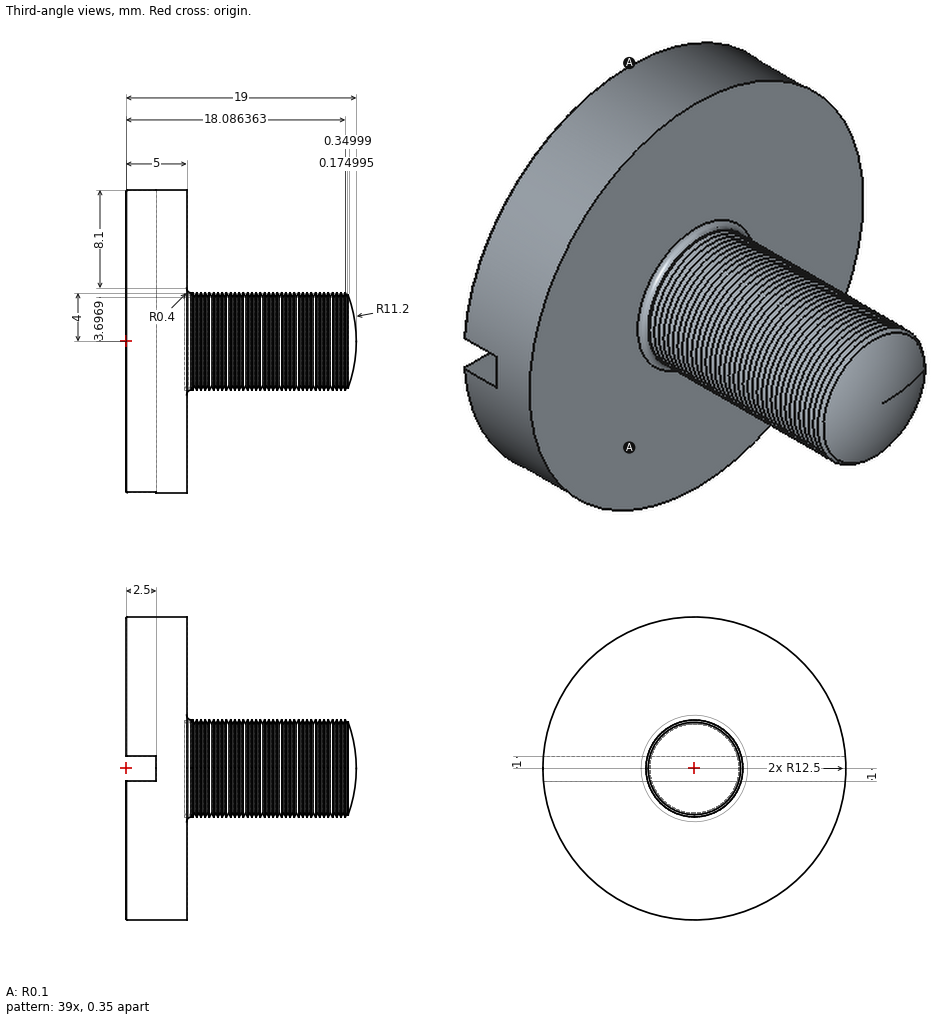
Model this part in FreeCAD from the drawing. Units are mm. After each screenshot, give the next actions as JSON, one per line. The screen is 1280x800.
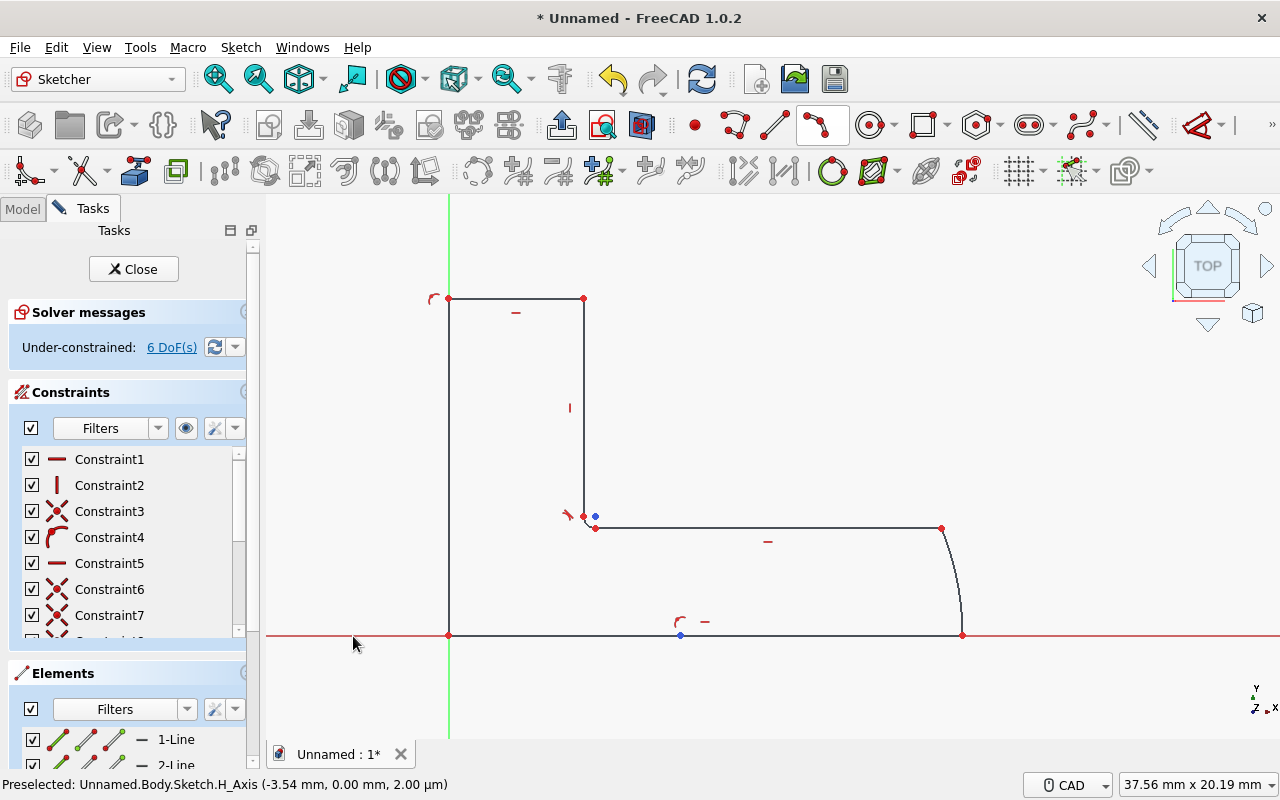
{"action": "scroll", "coordinate": [587, 525], "scroll_direction": "up", "scroll_amount": 7}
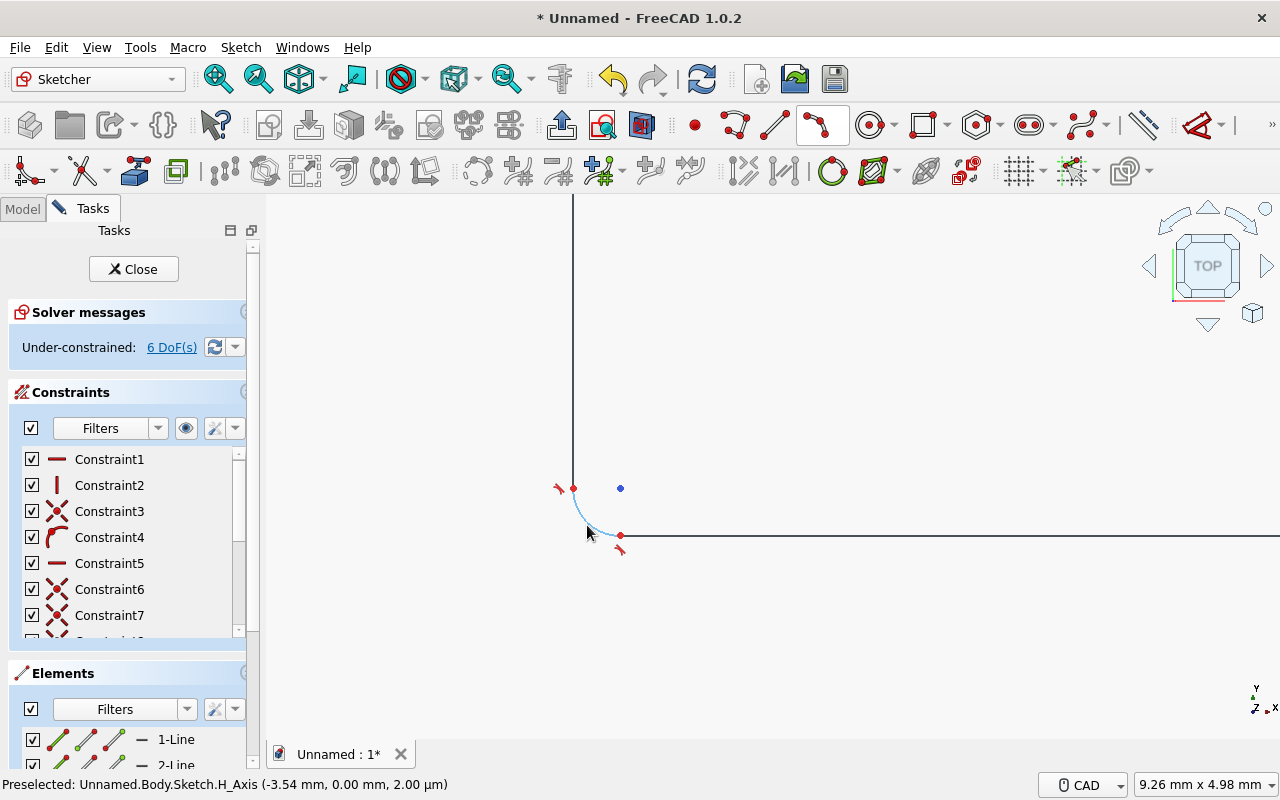
{"action": "left_click", "coordinate": [587, 522]}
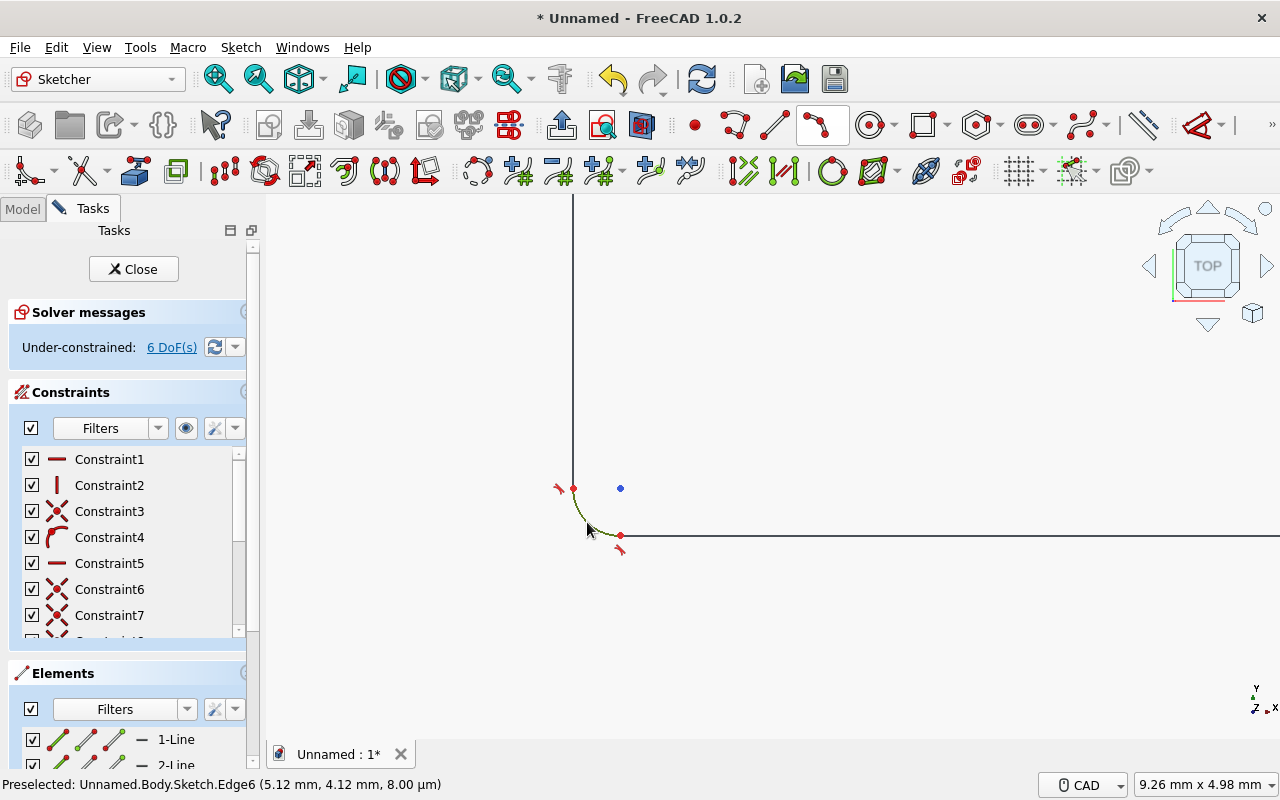
{"action": "left_click", "coordinate": [1224, 126]}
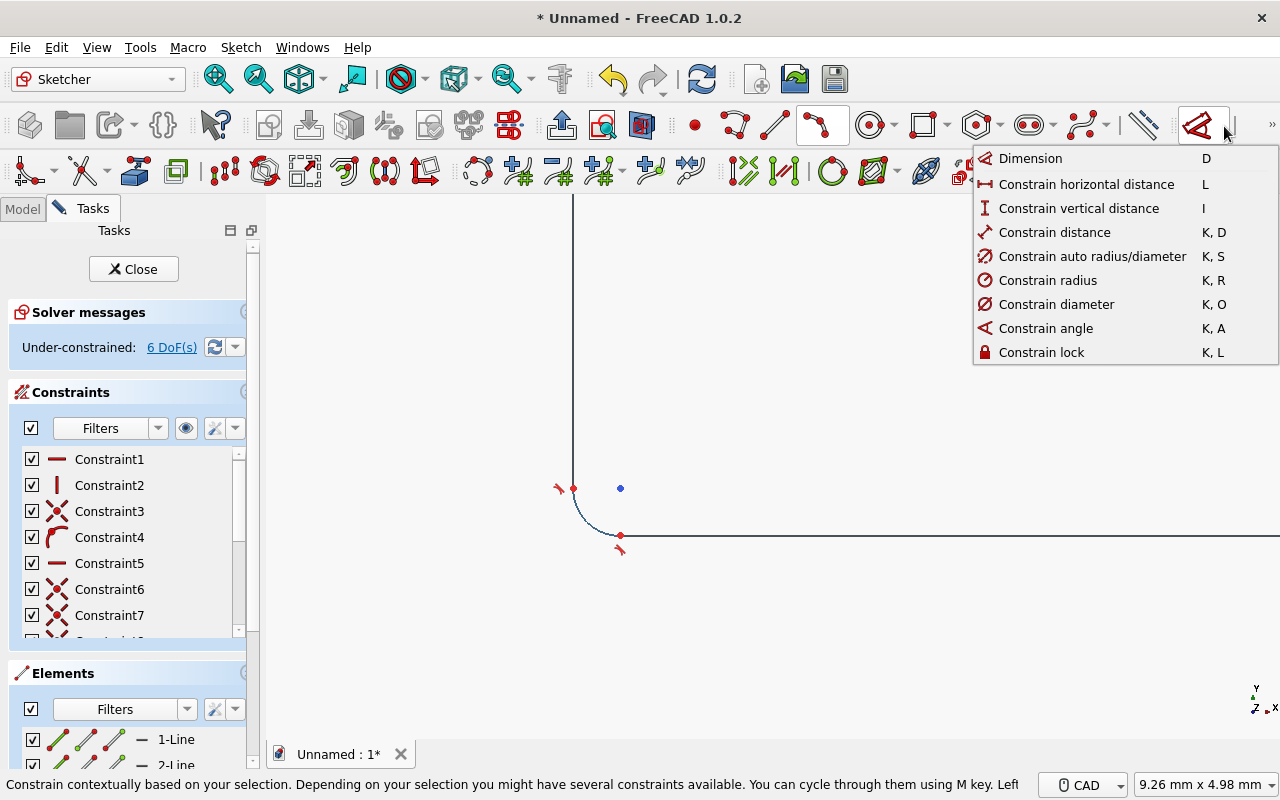
{"action": "left_click", "coordinate": [1126, 280]}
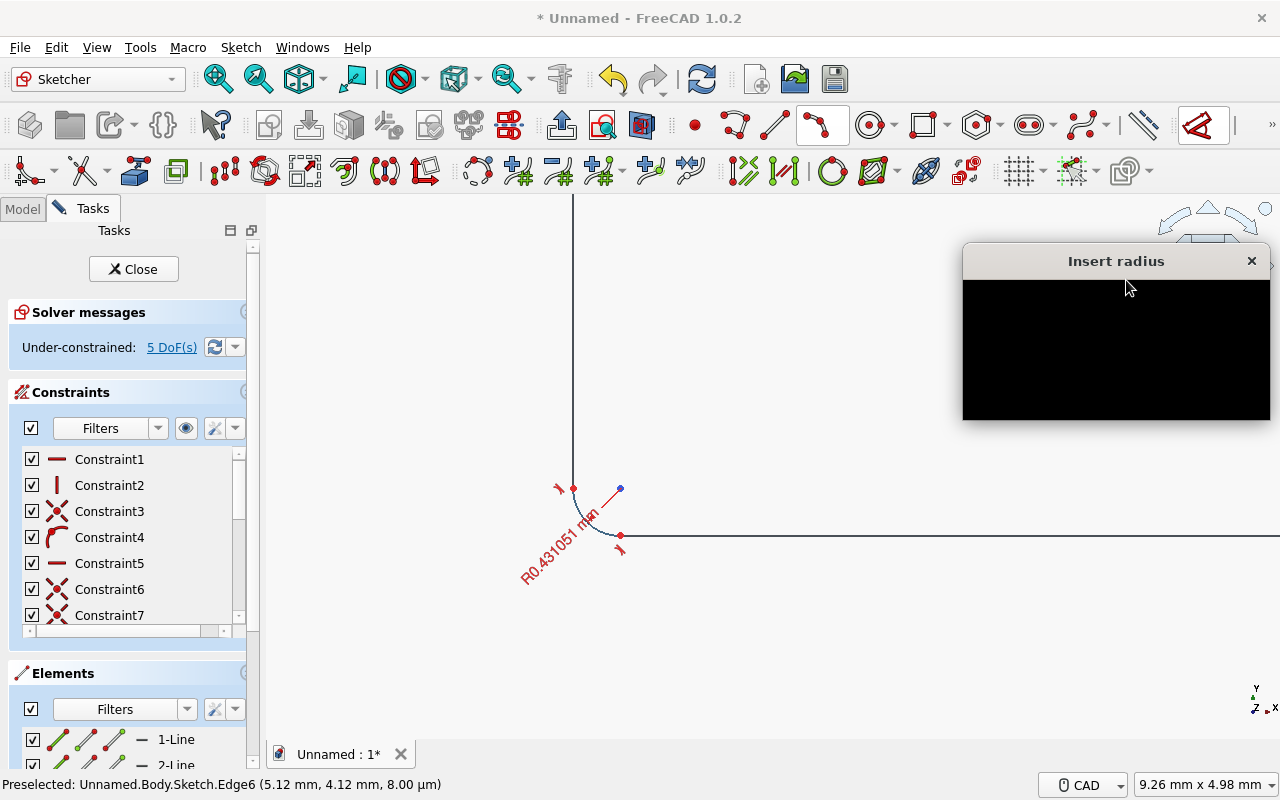
{"action": "type", "text": "0.4"}
{"action": "key", "text": "Return"}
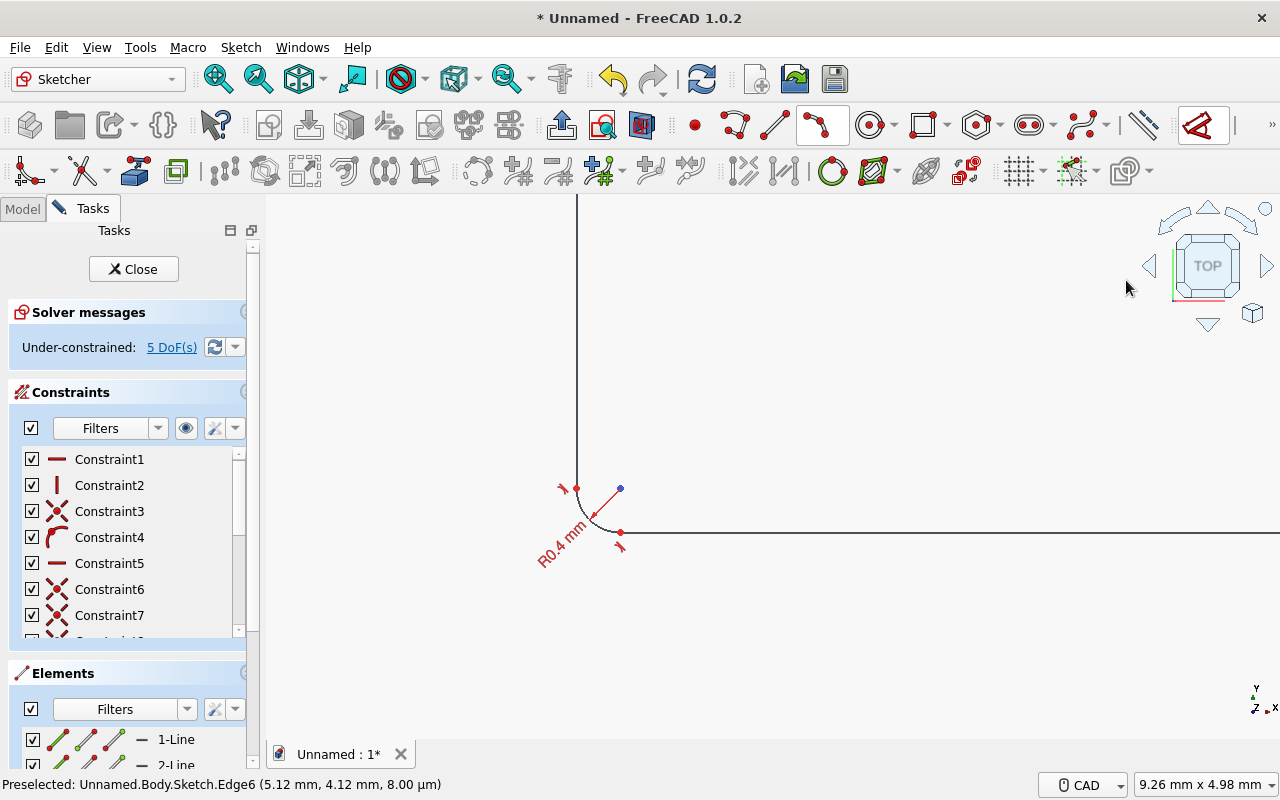
{"action": "scroll", "coordinate": [587, 525], "scroll_direction": "down", "scroll_amount": 7}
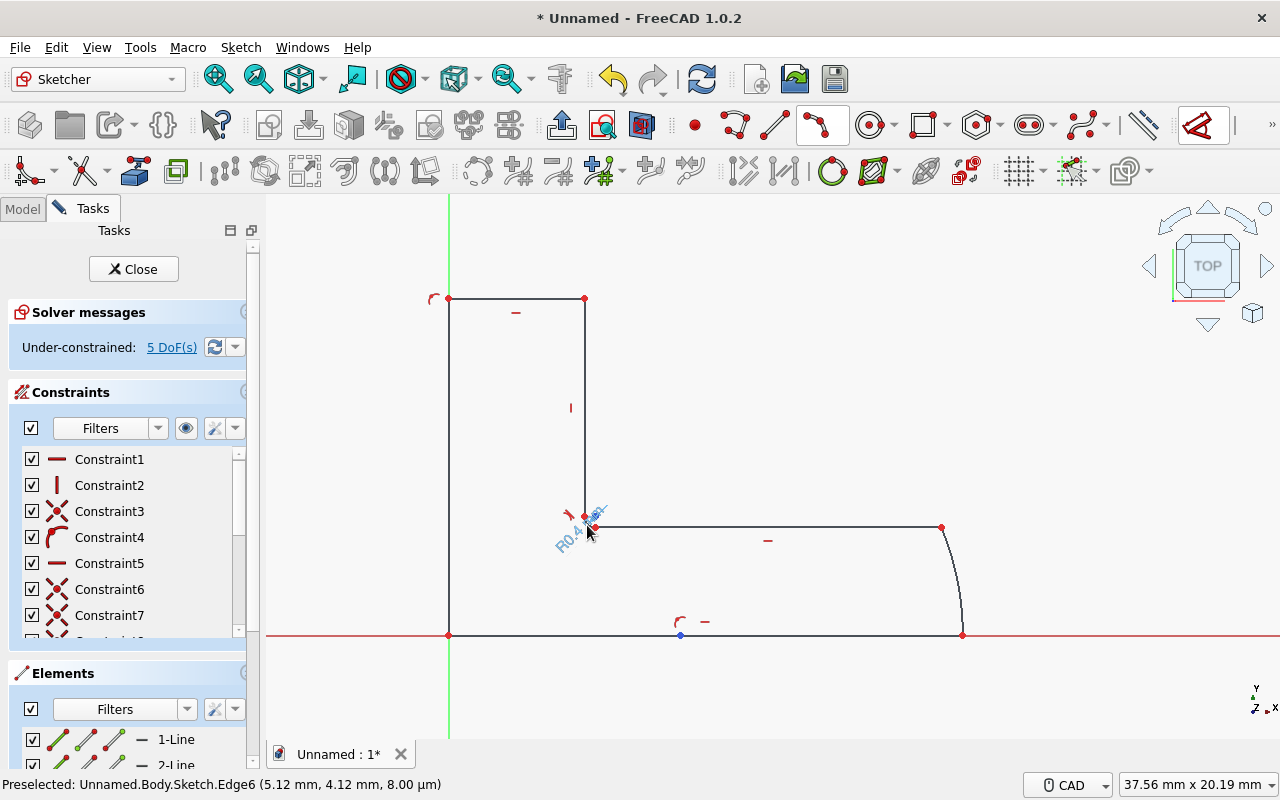
{"action": "left_click", "coordinate": [961, 602]}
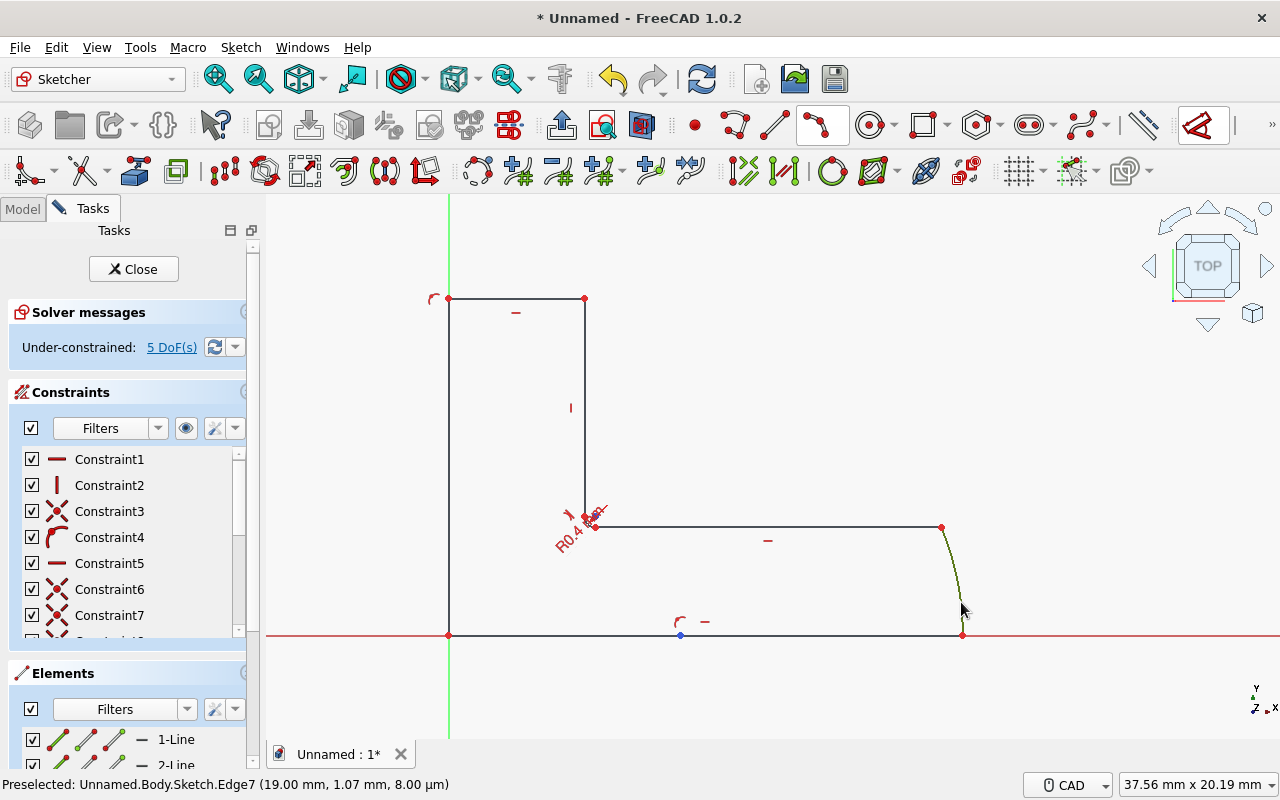
{"action": "key", "text": "k r"}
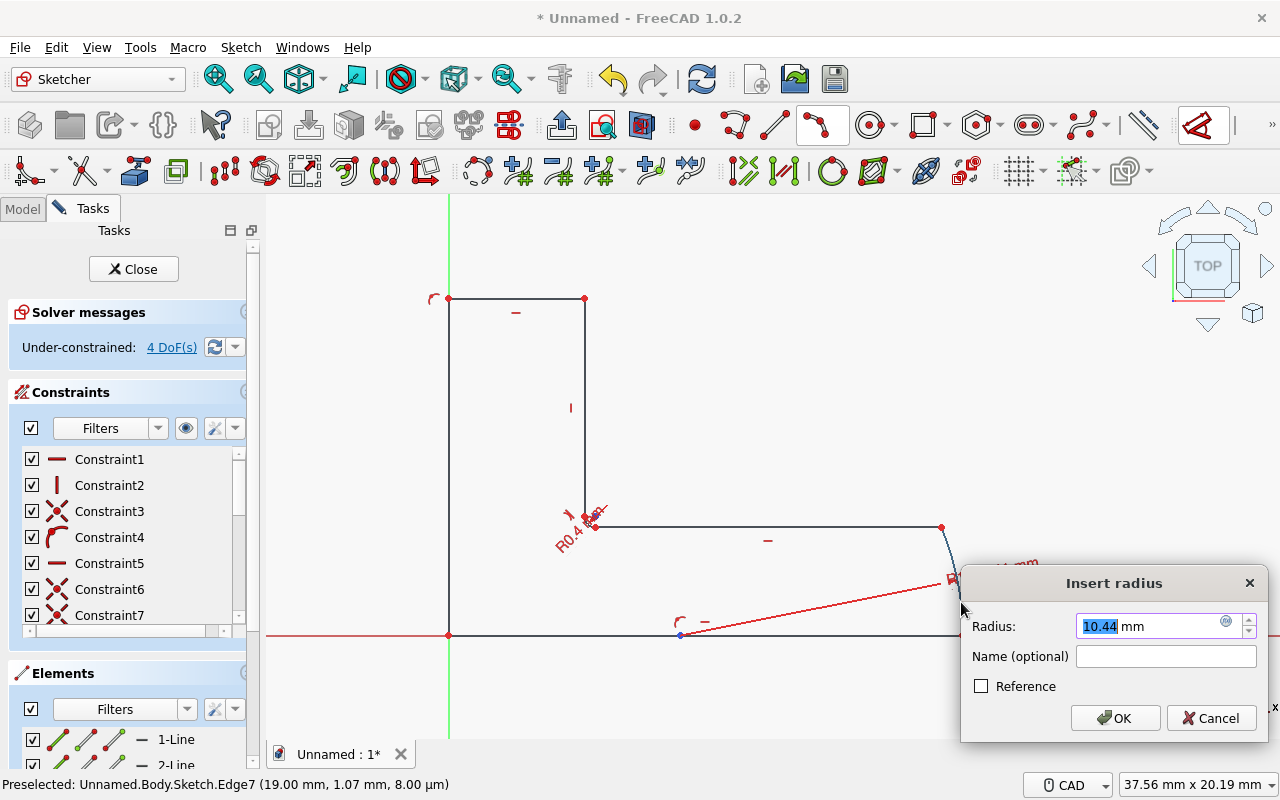
{"action": "type", "text": "11.2"}
{"action": "key", "text": "Return"}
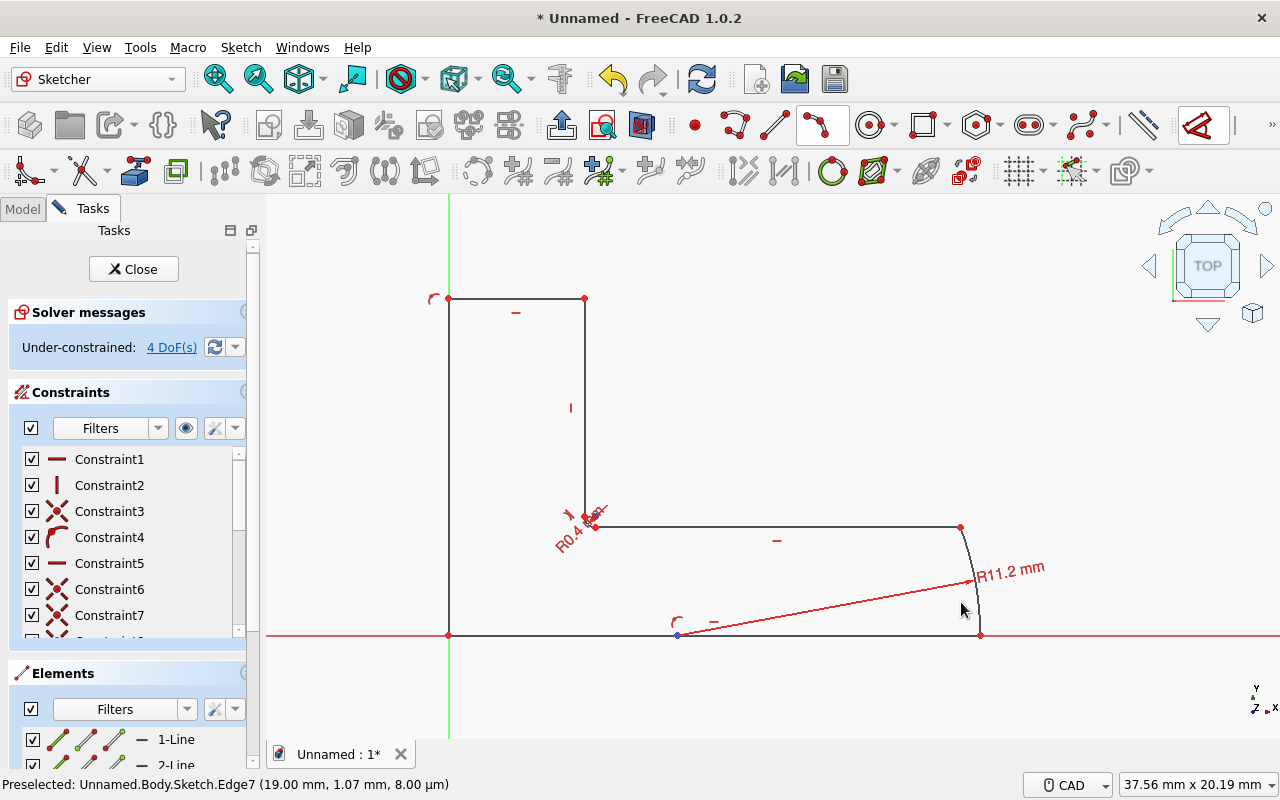
{"action": "left_click", "coordinate": [544, 299]}